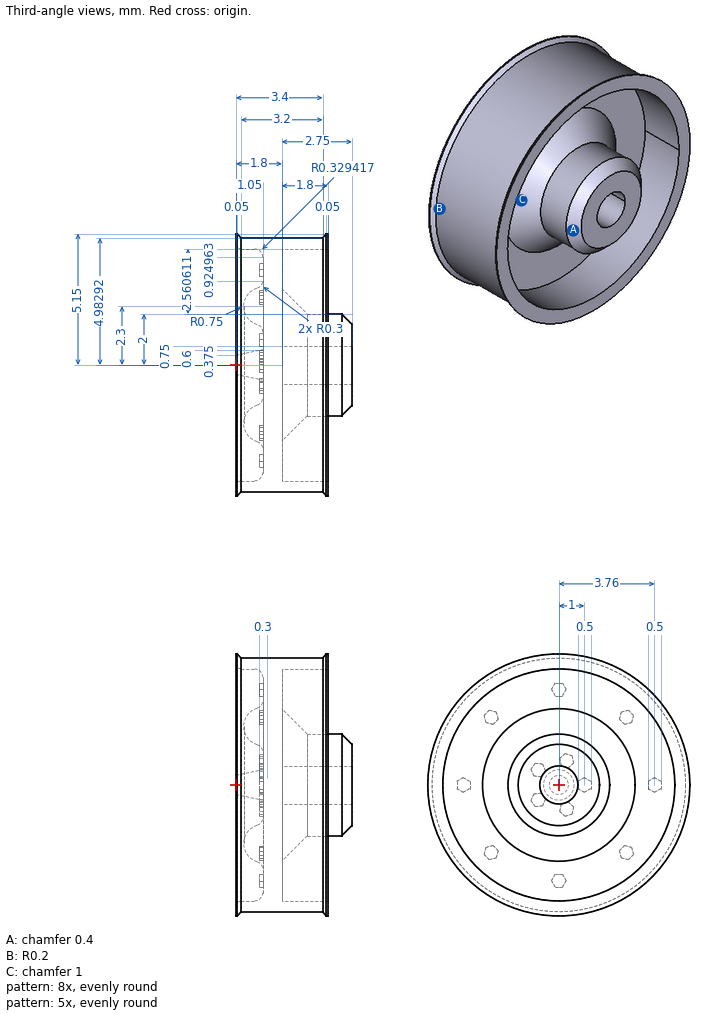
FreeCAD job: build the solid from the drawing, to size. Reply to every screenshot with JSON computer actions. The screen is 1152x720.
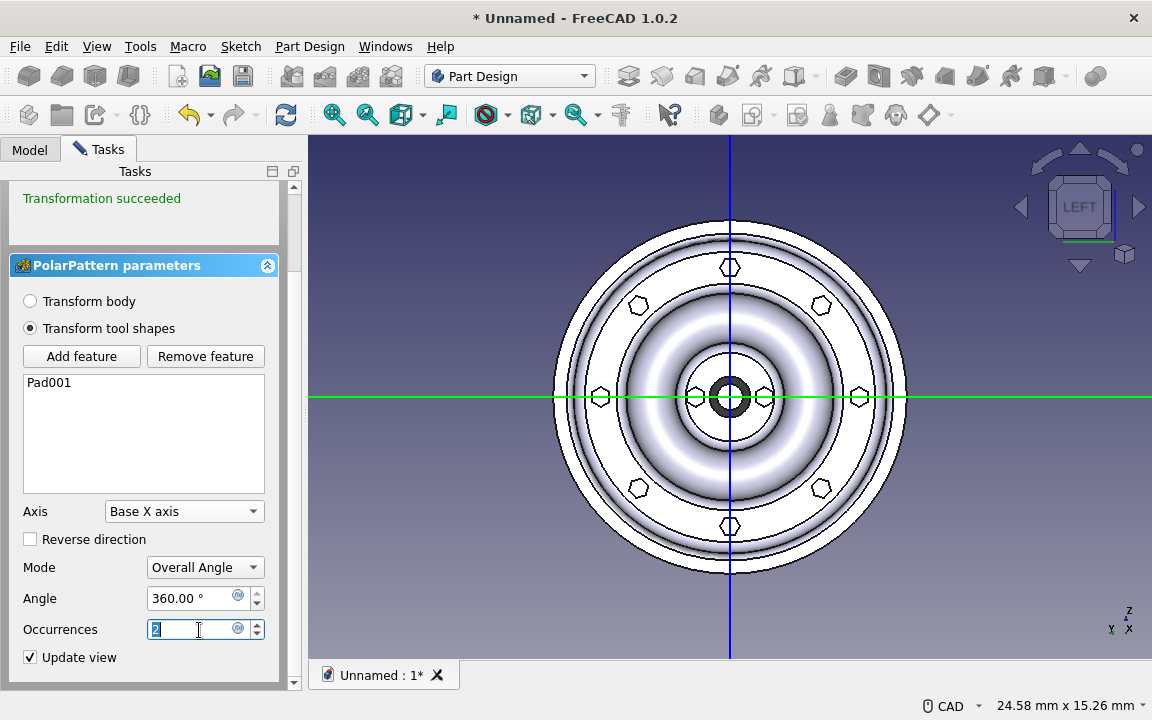
{"action": "type", "text": "5"}
{"action": "key", "text": "Tab"}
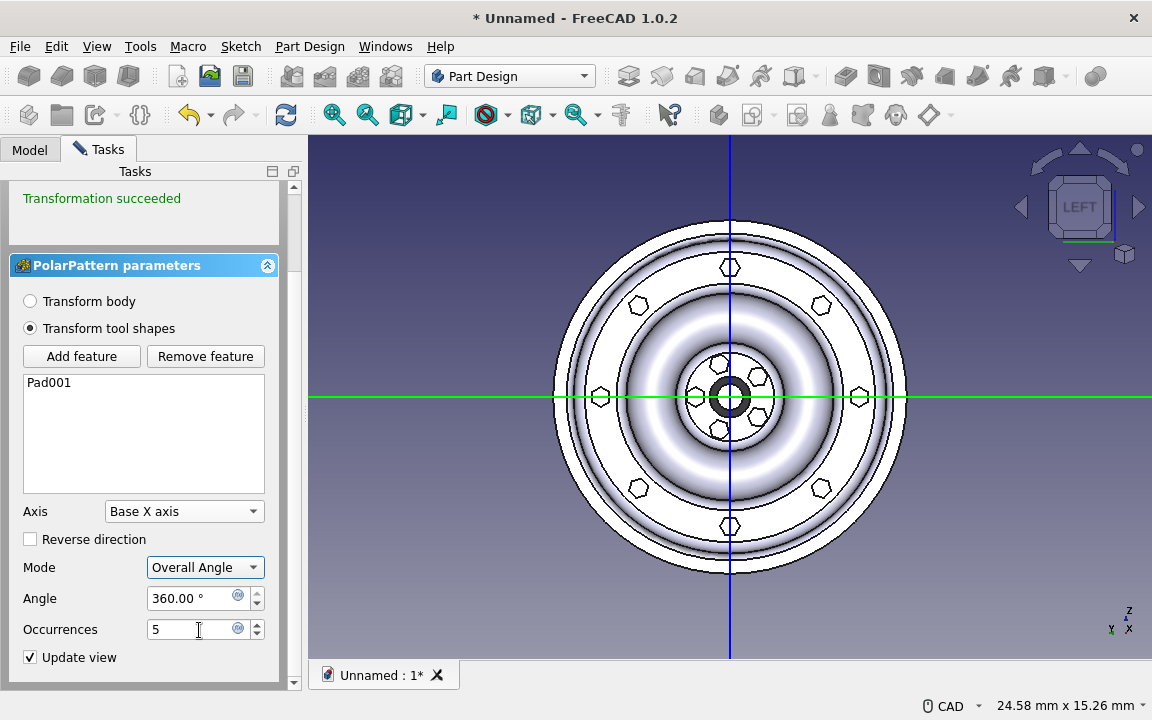
{"action": "scroll", "coordinate": [294, 436], "scroll_direction": "up", "scroll_amount": 3}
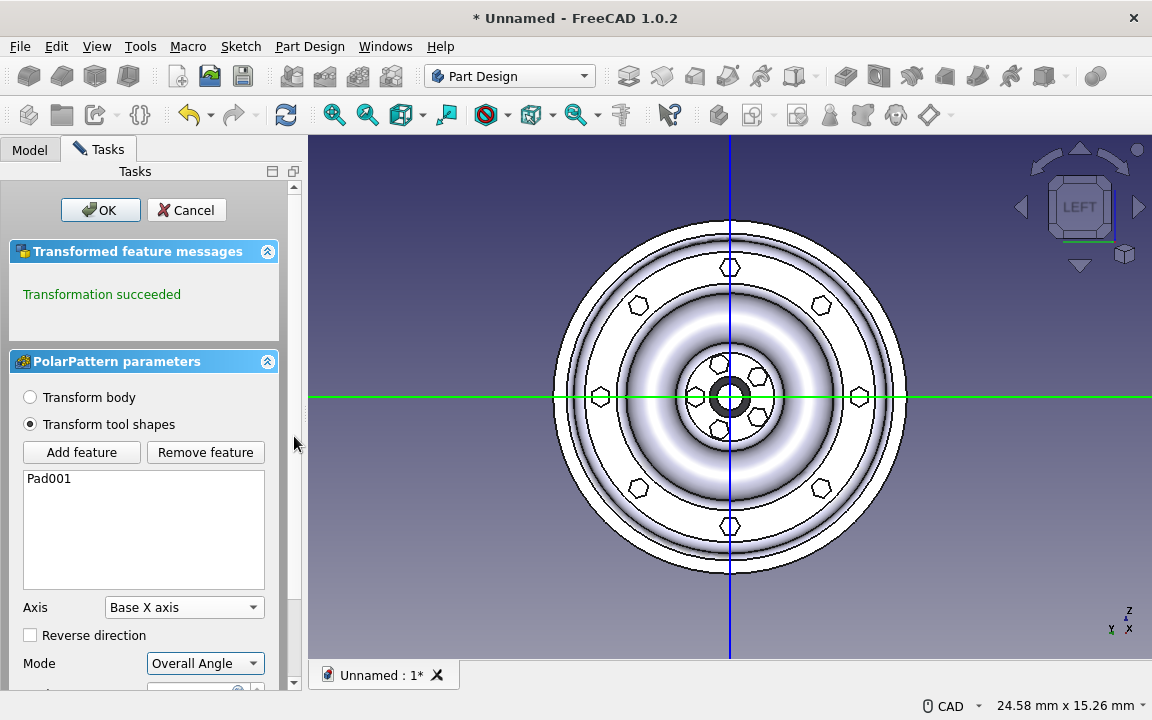
{"action": "left_click", "coordinate": [101, 210]}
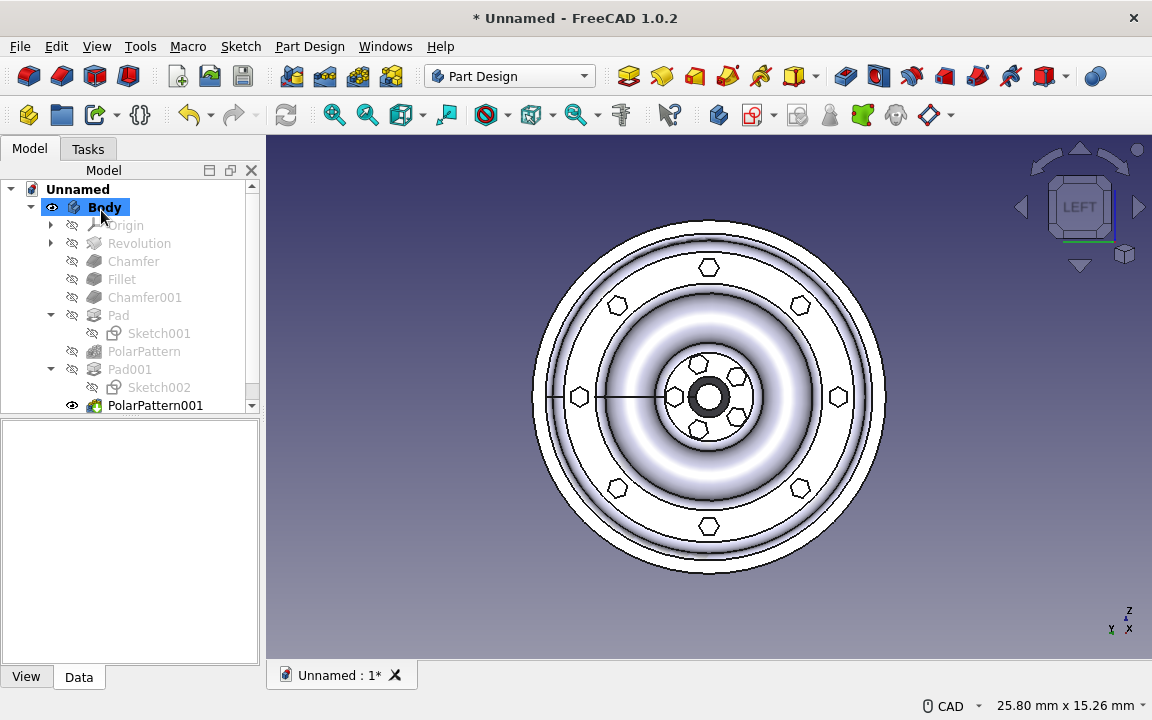
{"action": "key", "text": "0"}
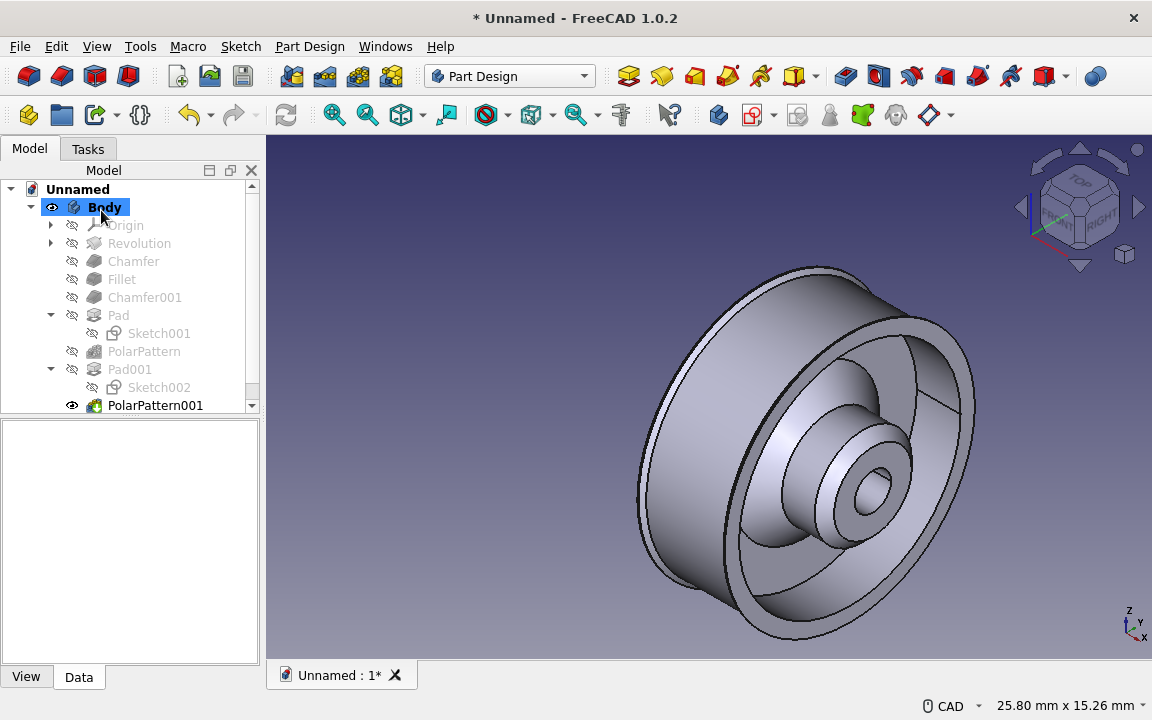
{"action": "left_click", "coordinate": [335, 116]}